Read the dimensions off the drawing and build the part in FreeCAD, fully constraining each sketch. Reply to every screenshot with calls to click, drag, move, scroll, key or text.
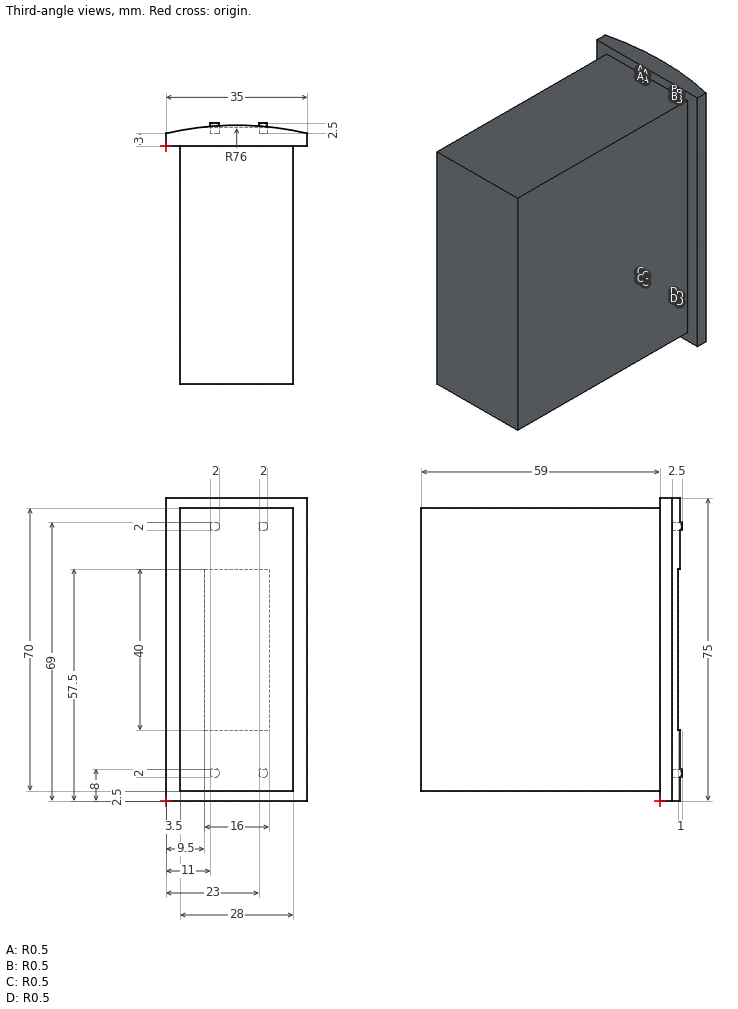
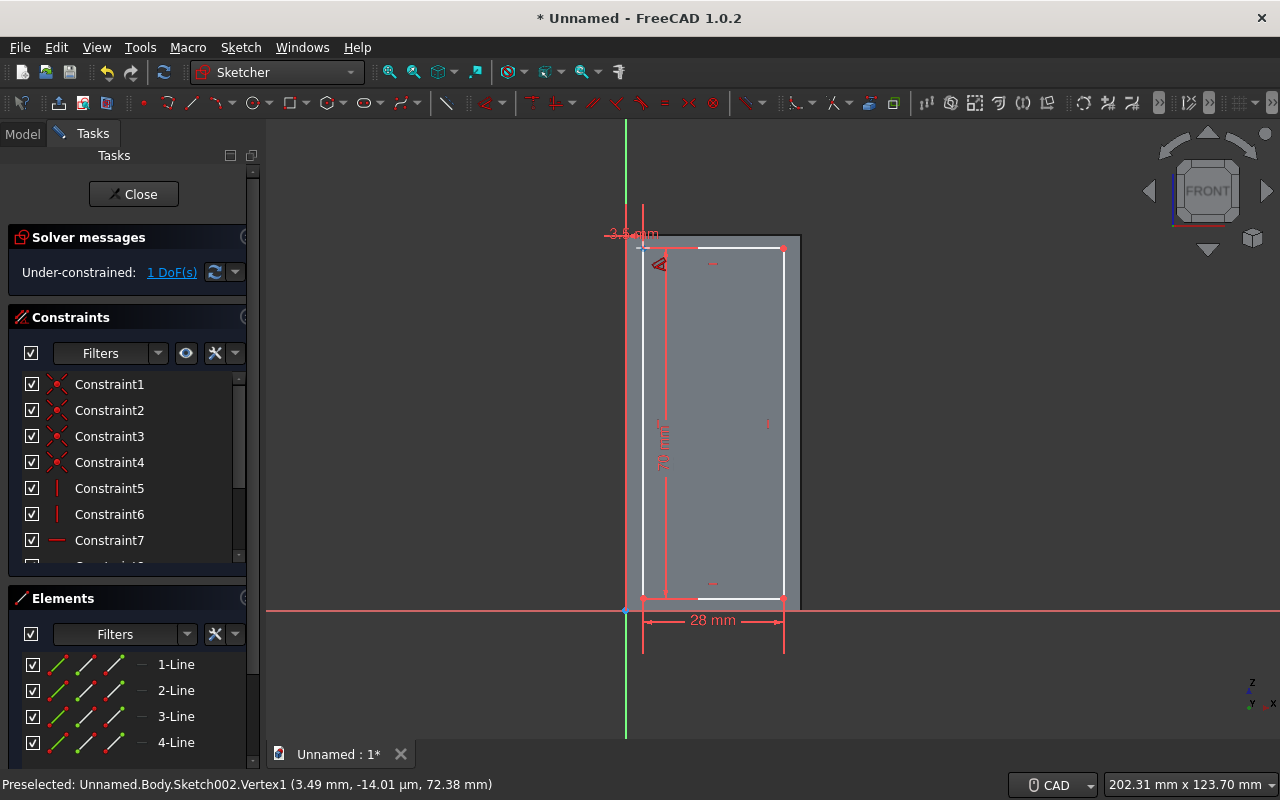
scroll(643, 599, up, 6)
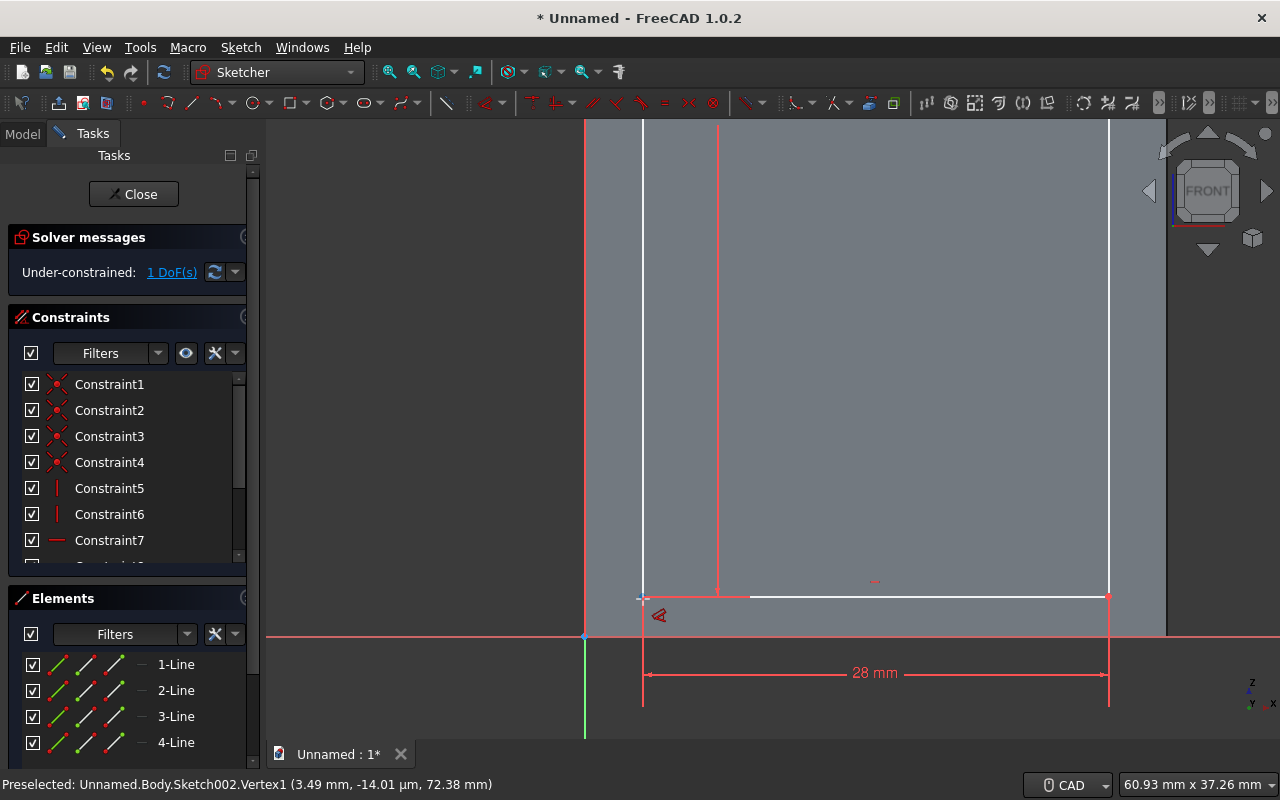
click(643, 597)
click(551, 617)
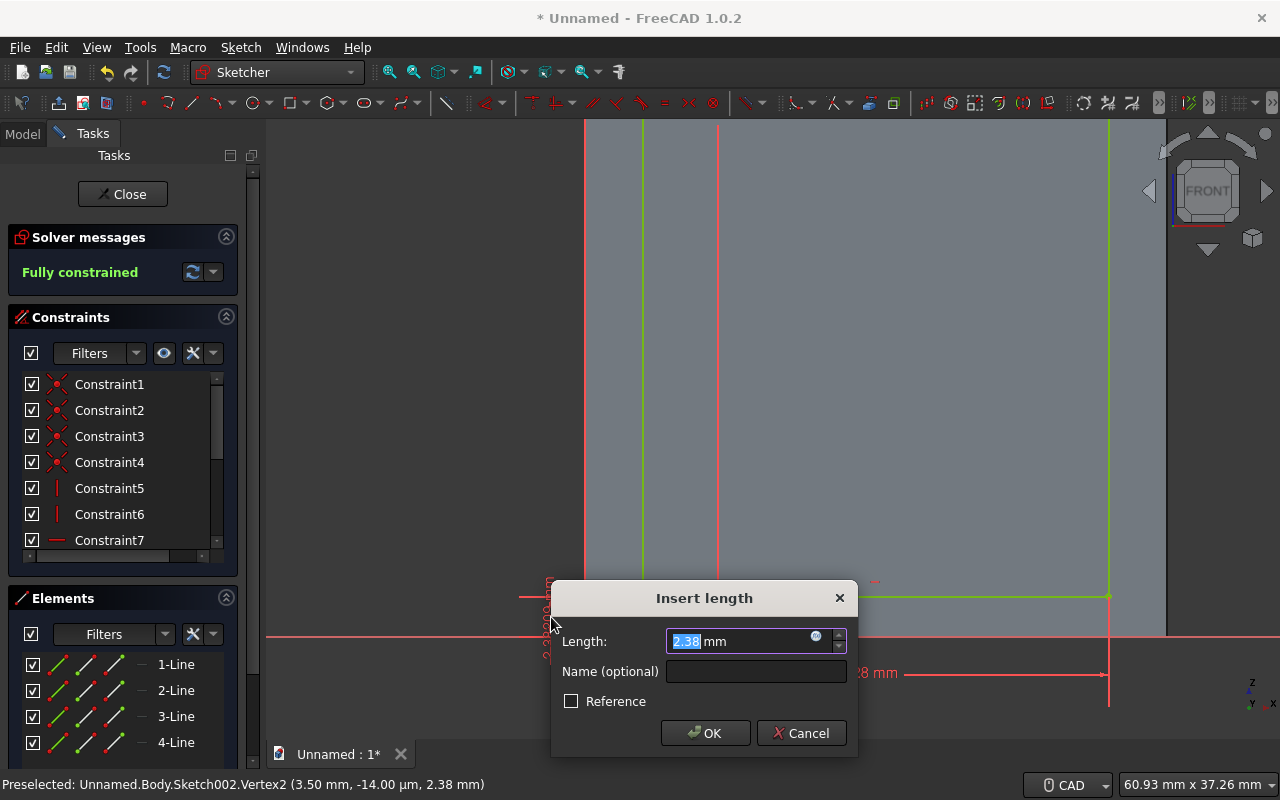
text(2.5)
key(Return)
key(Escape)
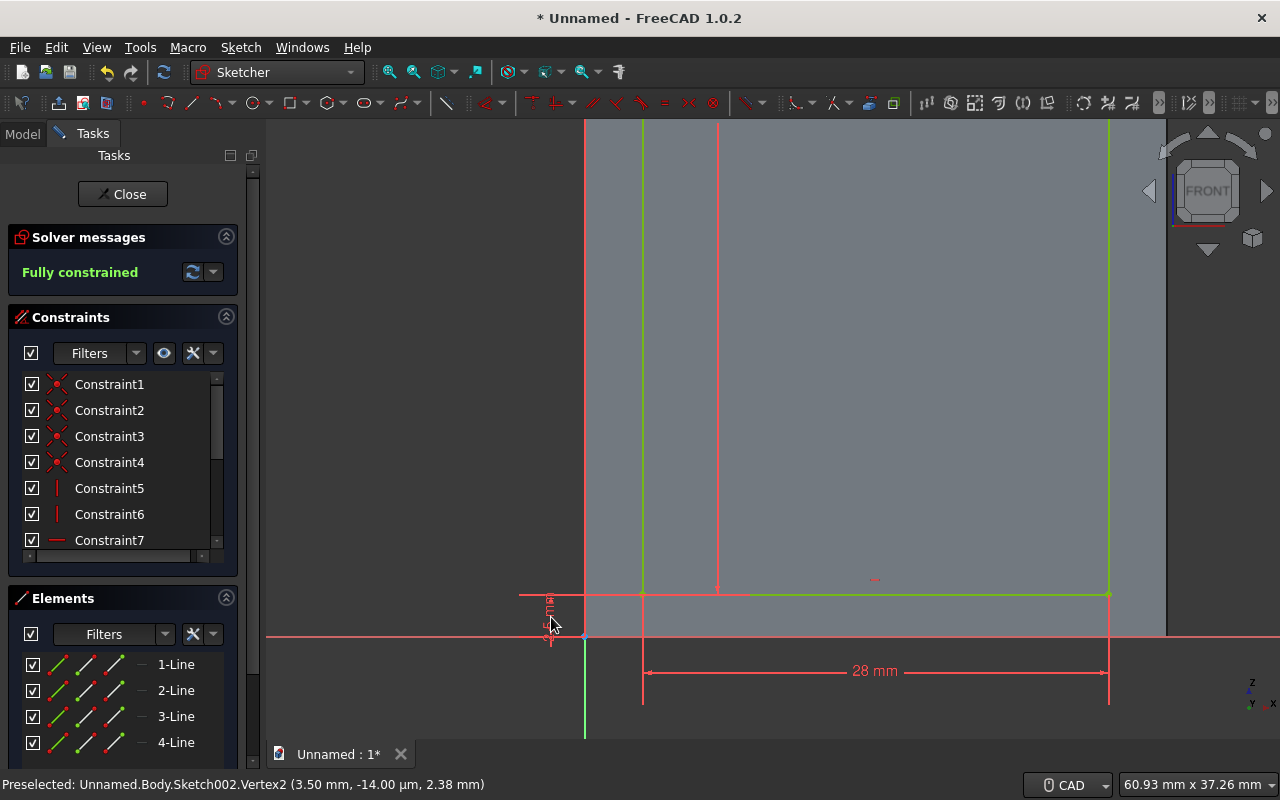
click(123, 194)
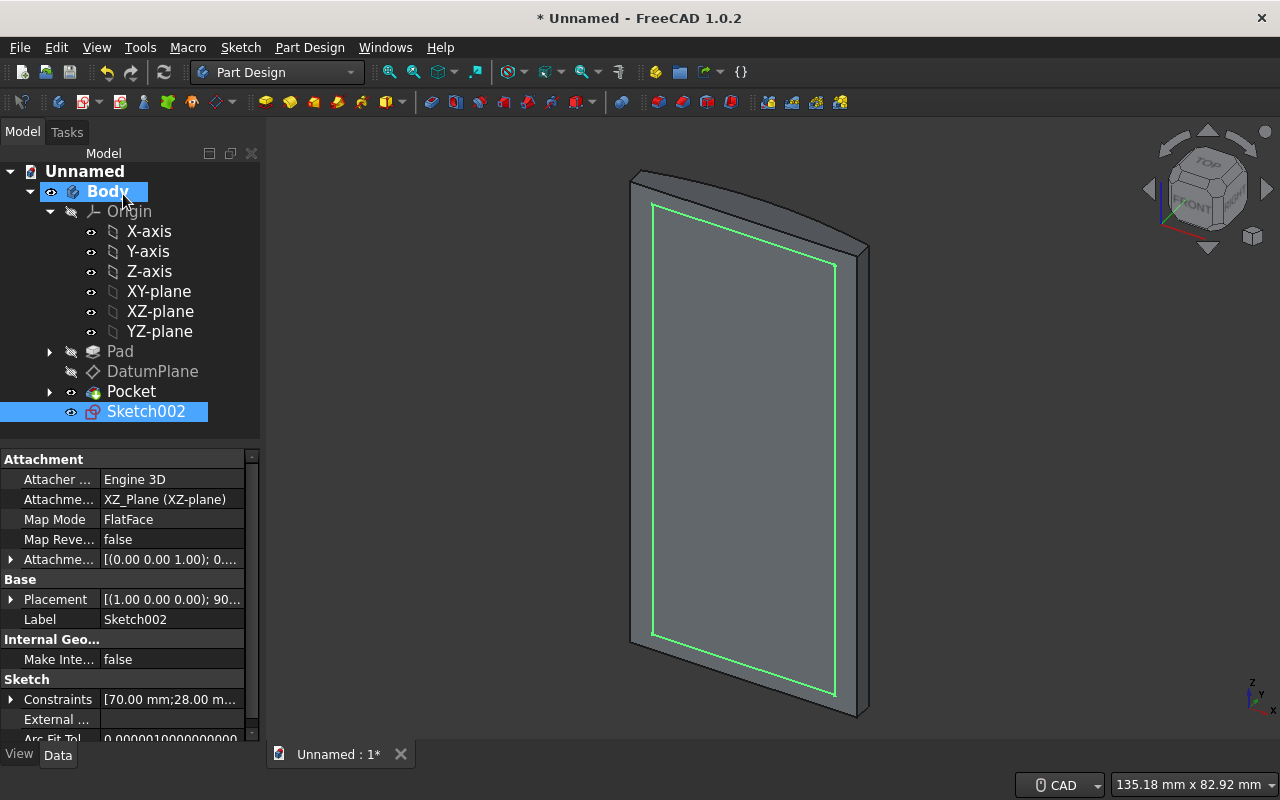
click(266, 102)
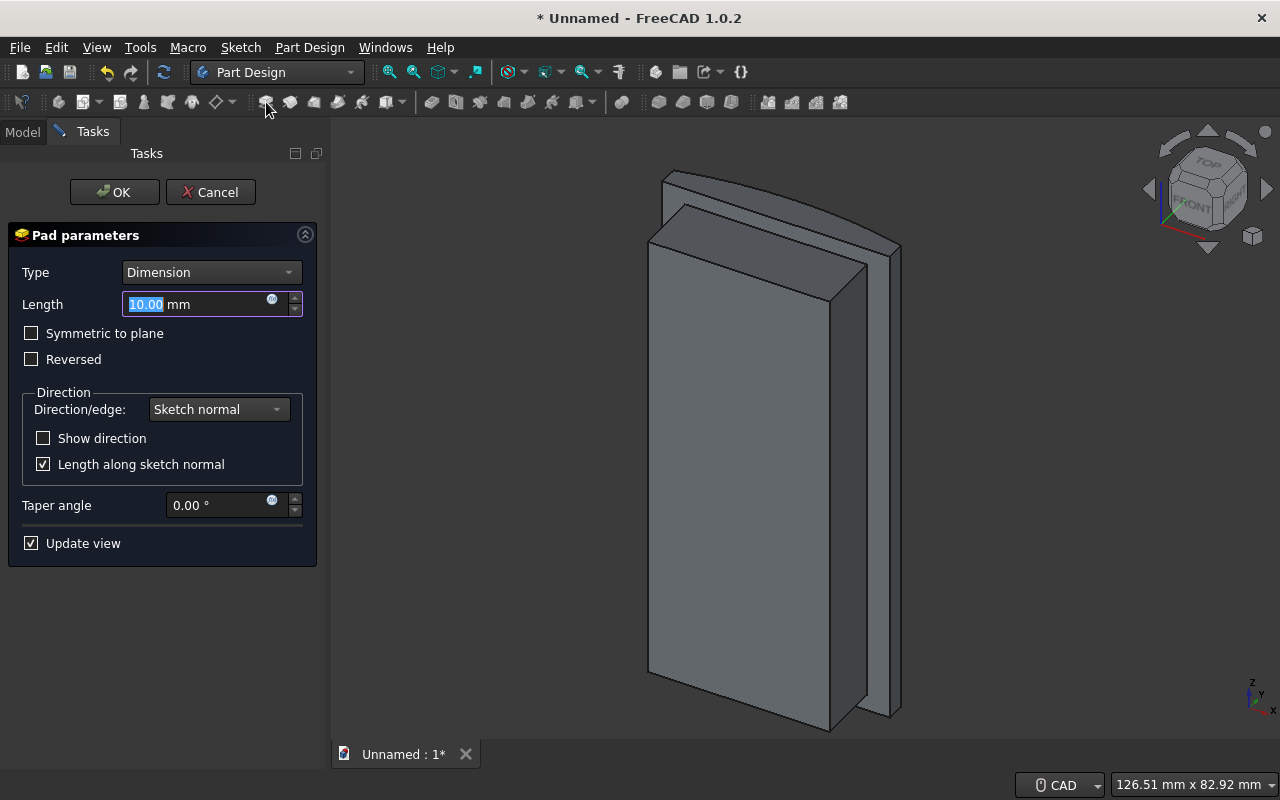
text(59)
key(Tab)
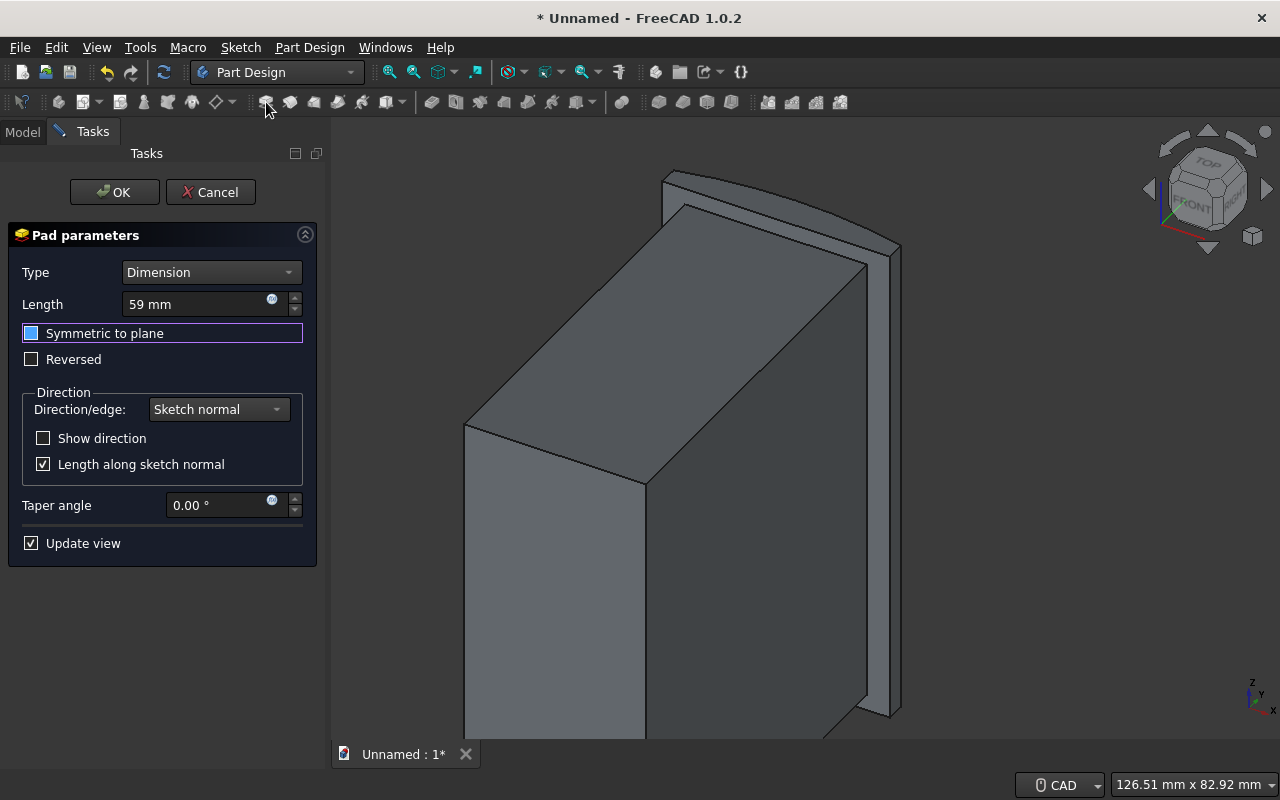
click(115, 192)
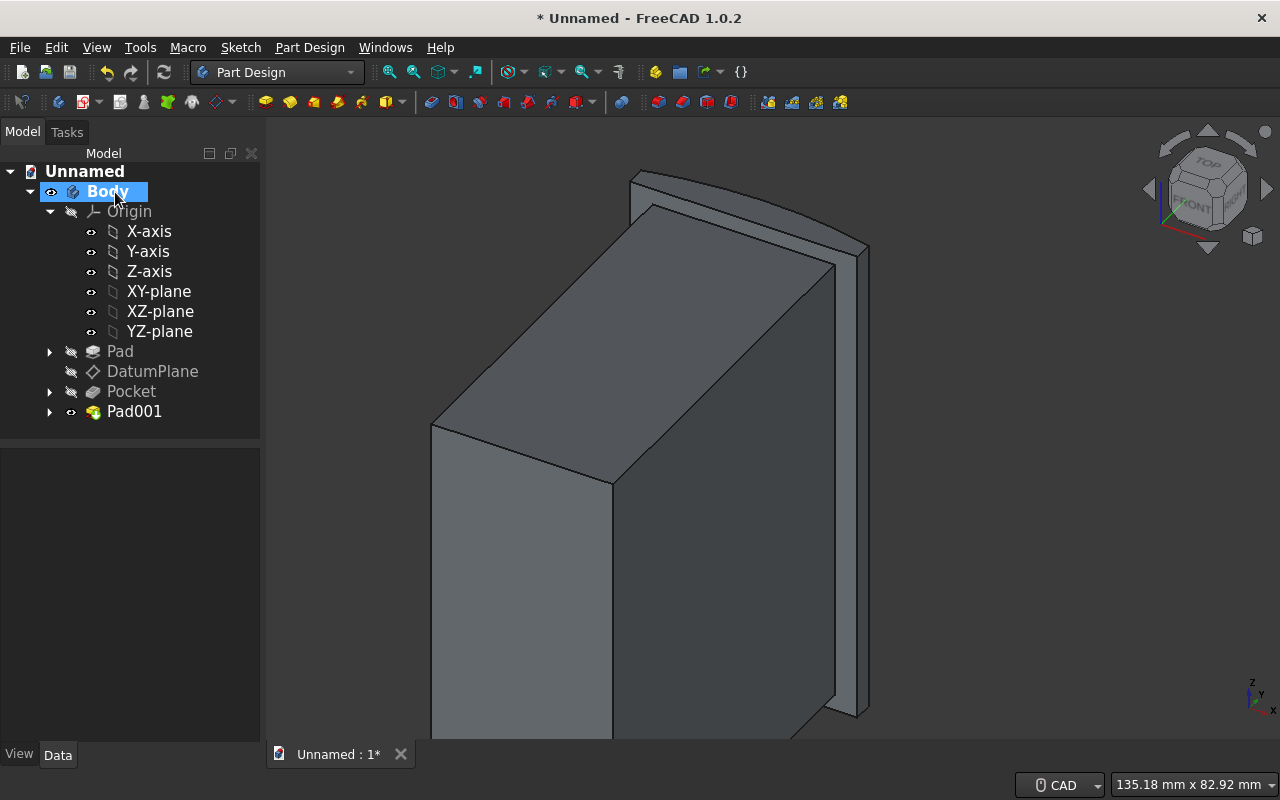
key(v)
key(f)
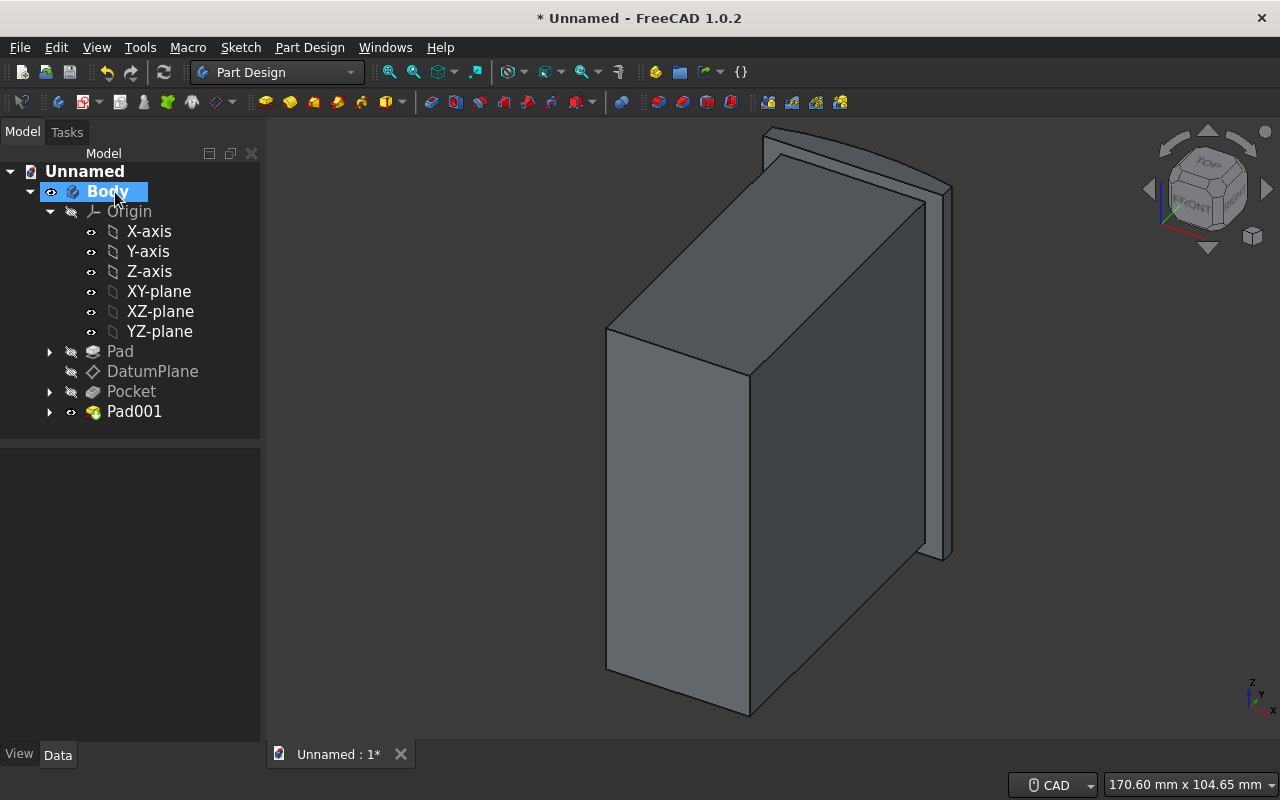
click(60, 102)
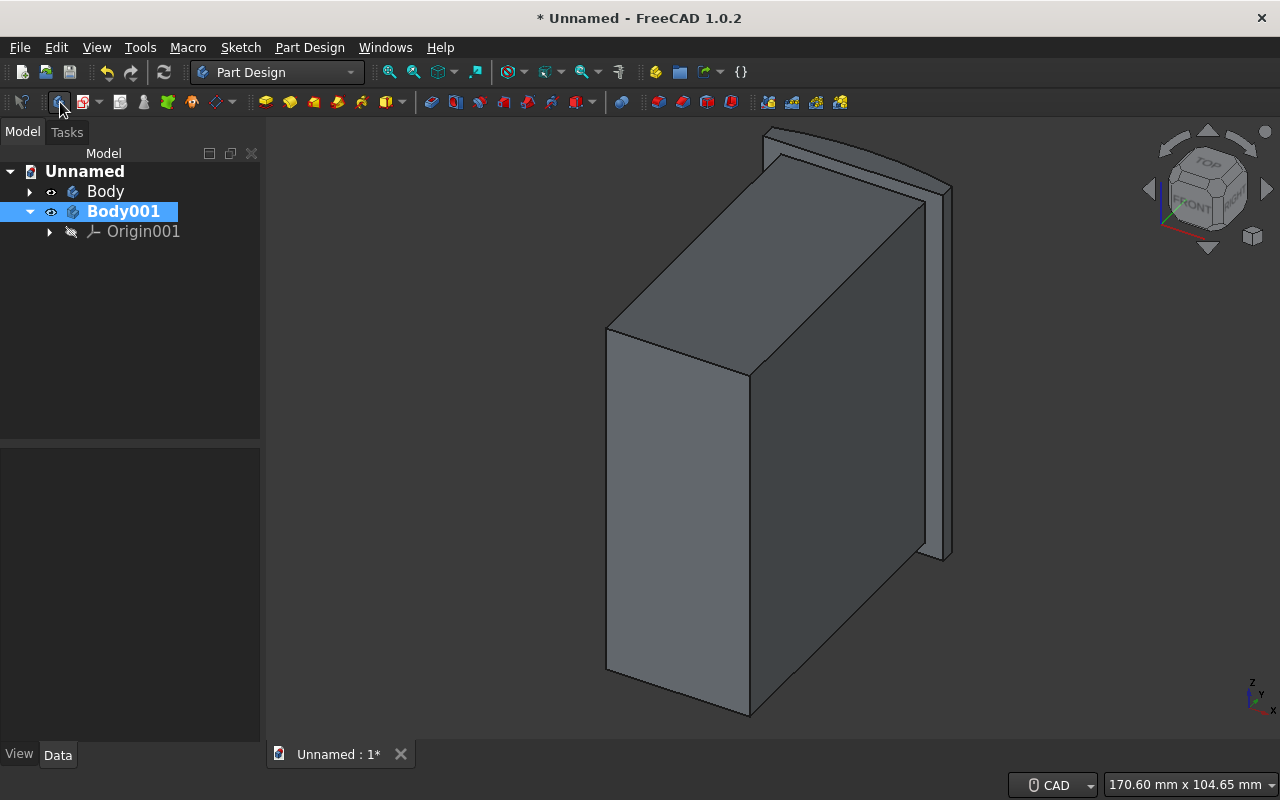
click(50, 232)